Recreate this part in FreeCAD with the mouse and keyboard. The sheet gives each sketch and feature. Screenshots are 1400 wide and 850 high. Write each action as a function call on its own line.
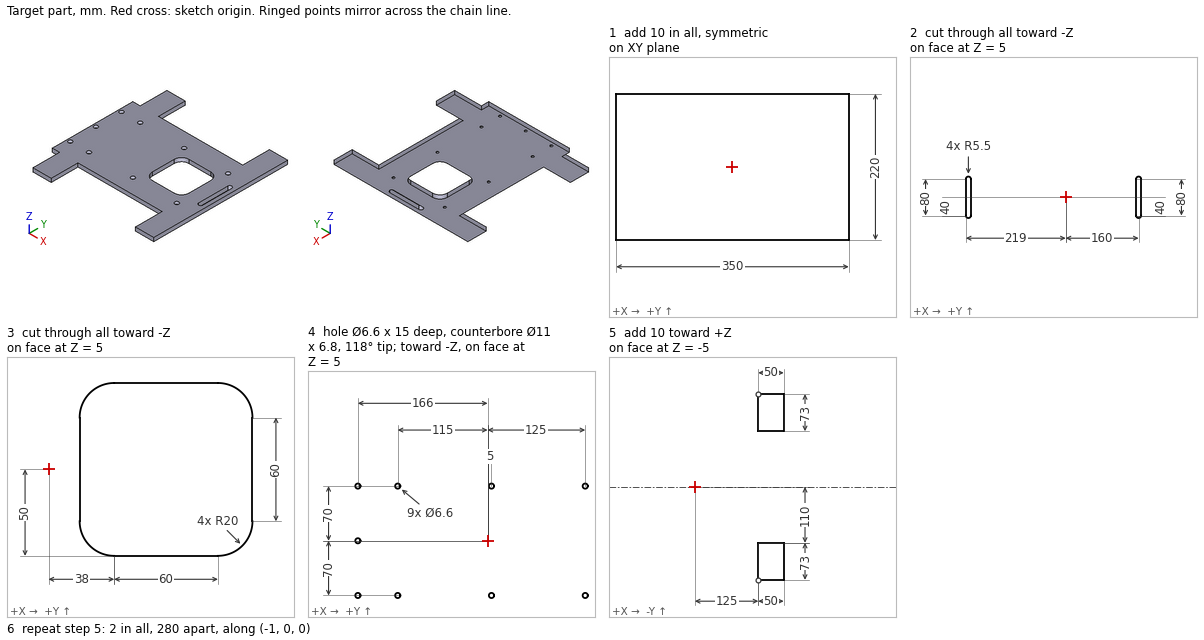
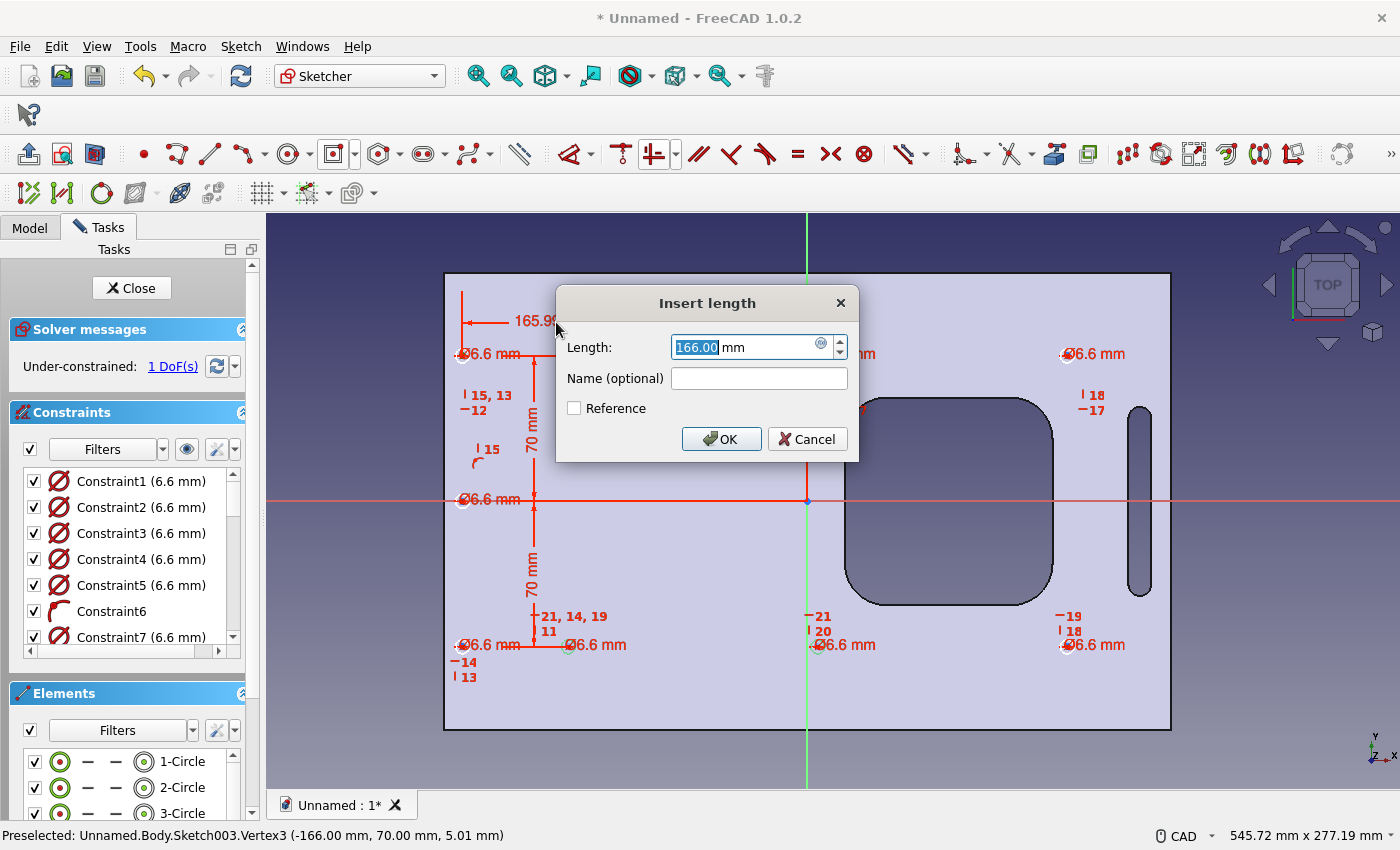
text(166)
key(Return)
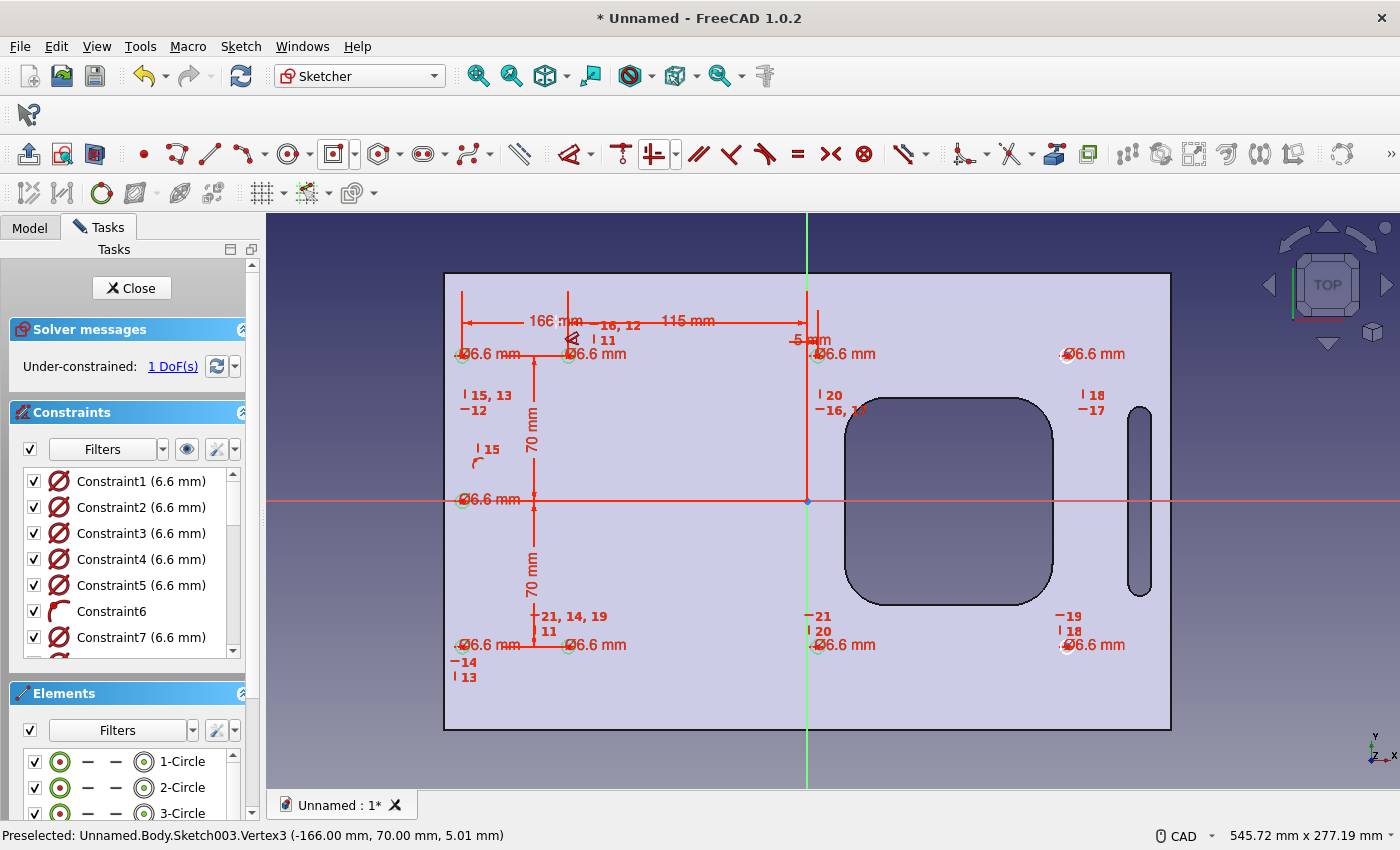
click(1067, 356)
click(937, 322)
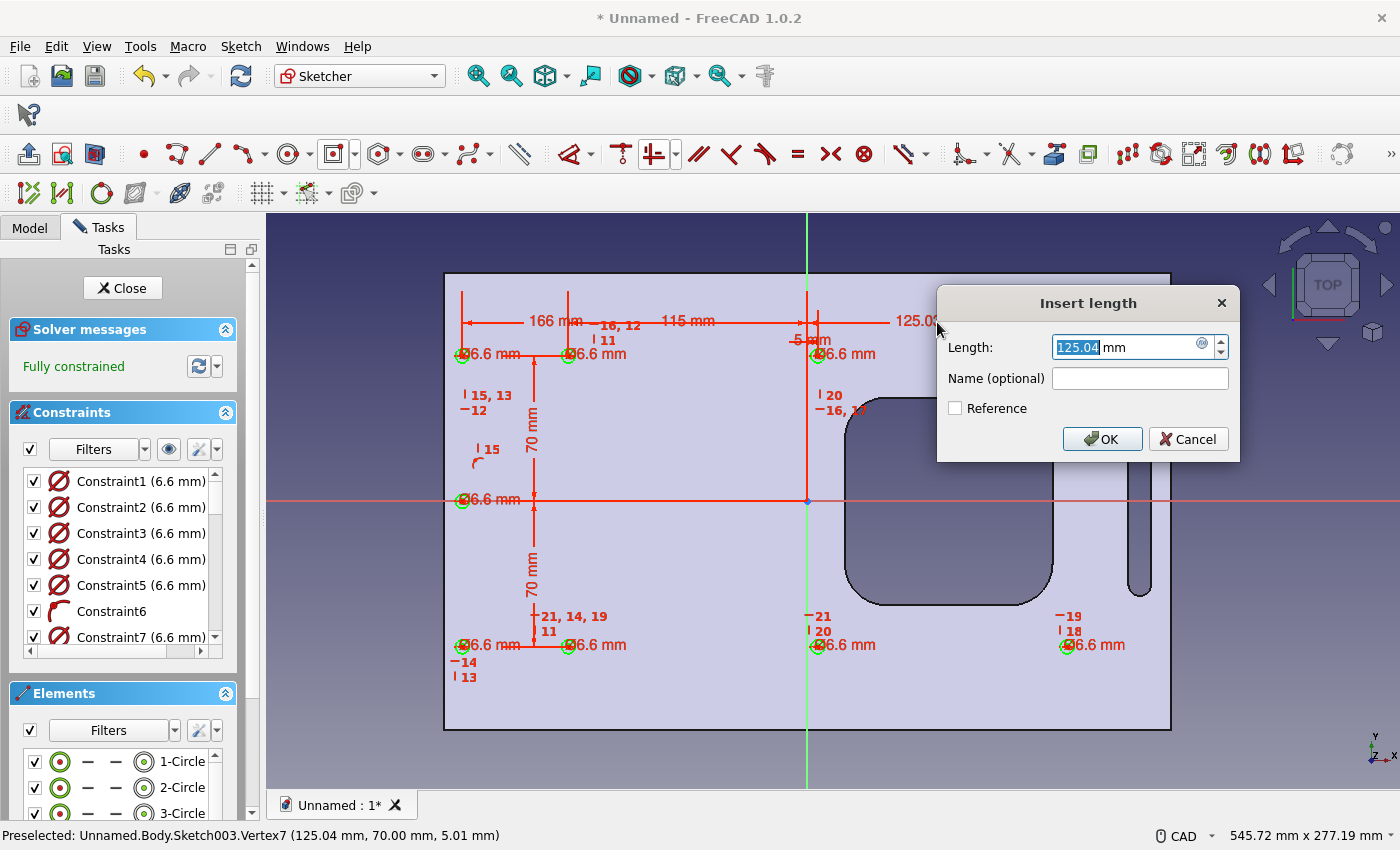
text(125)
key(Return)
key(Escape)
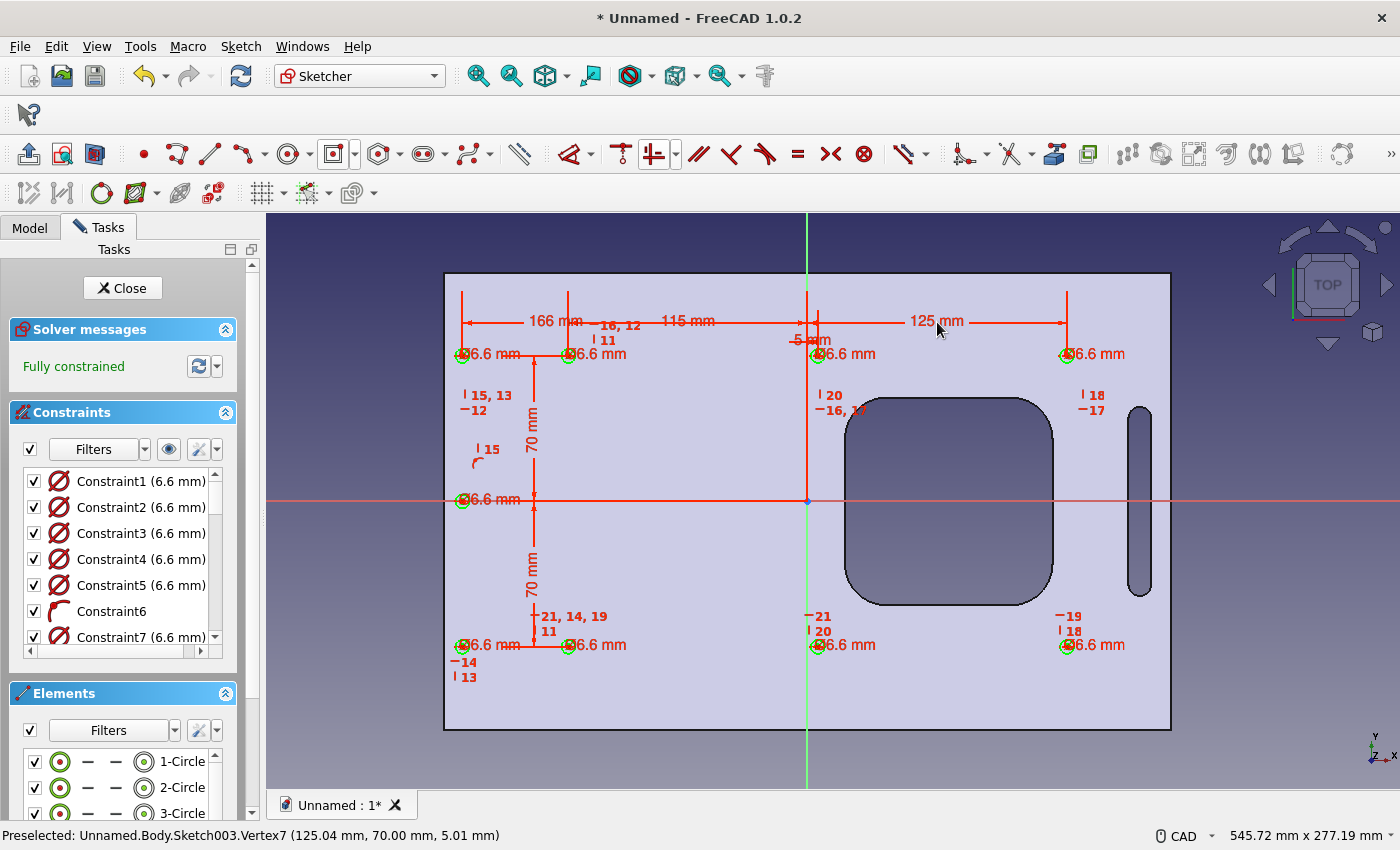
click(123, 288)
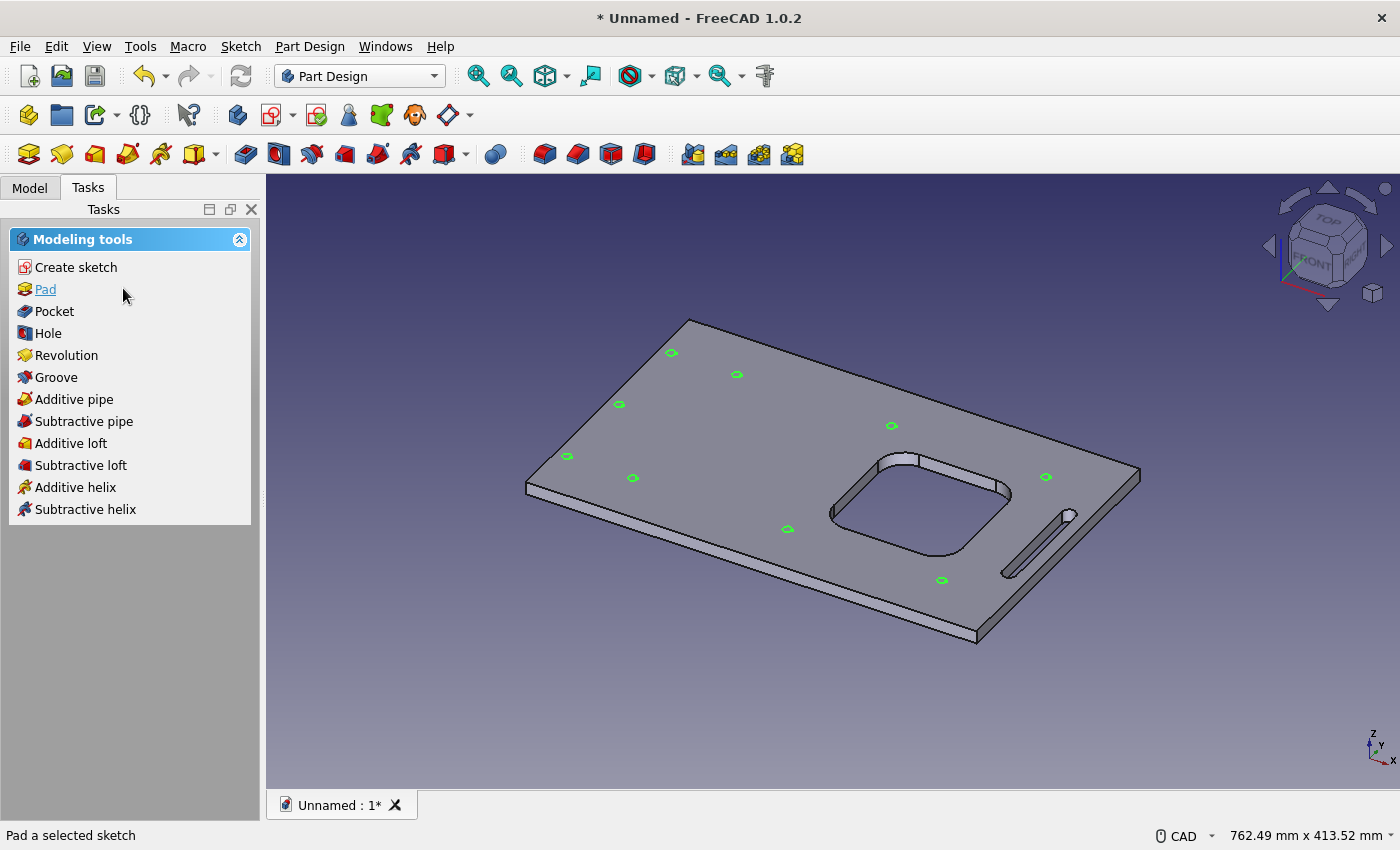
click(279, 154)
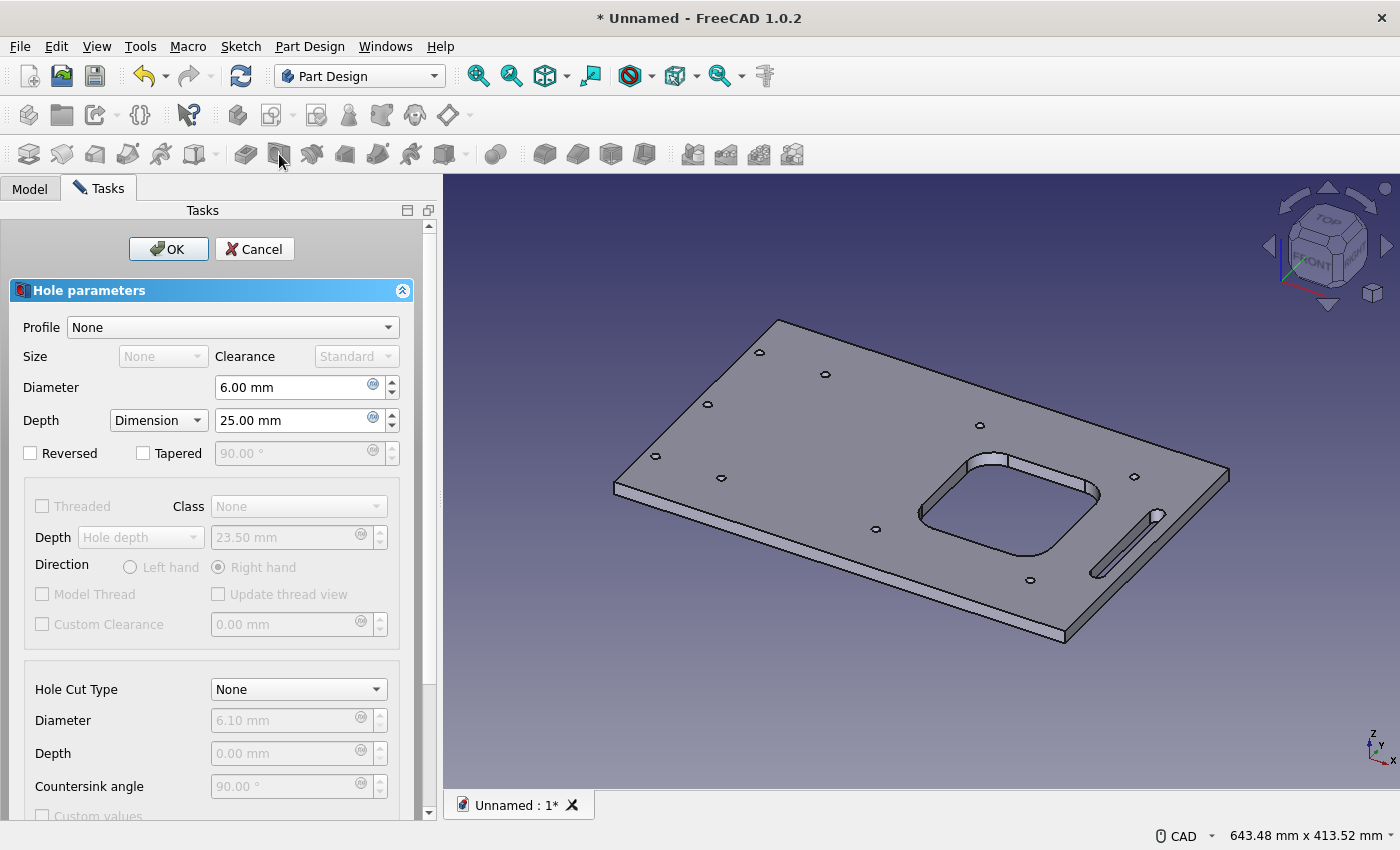
triple_click(300, 388)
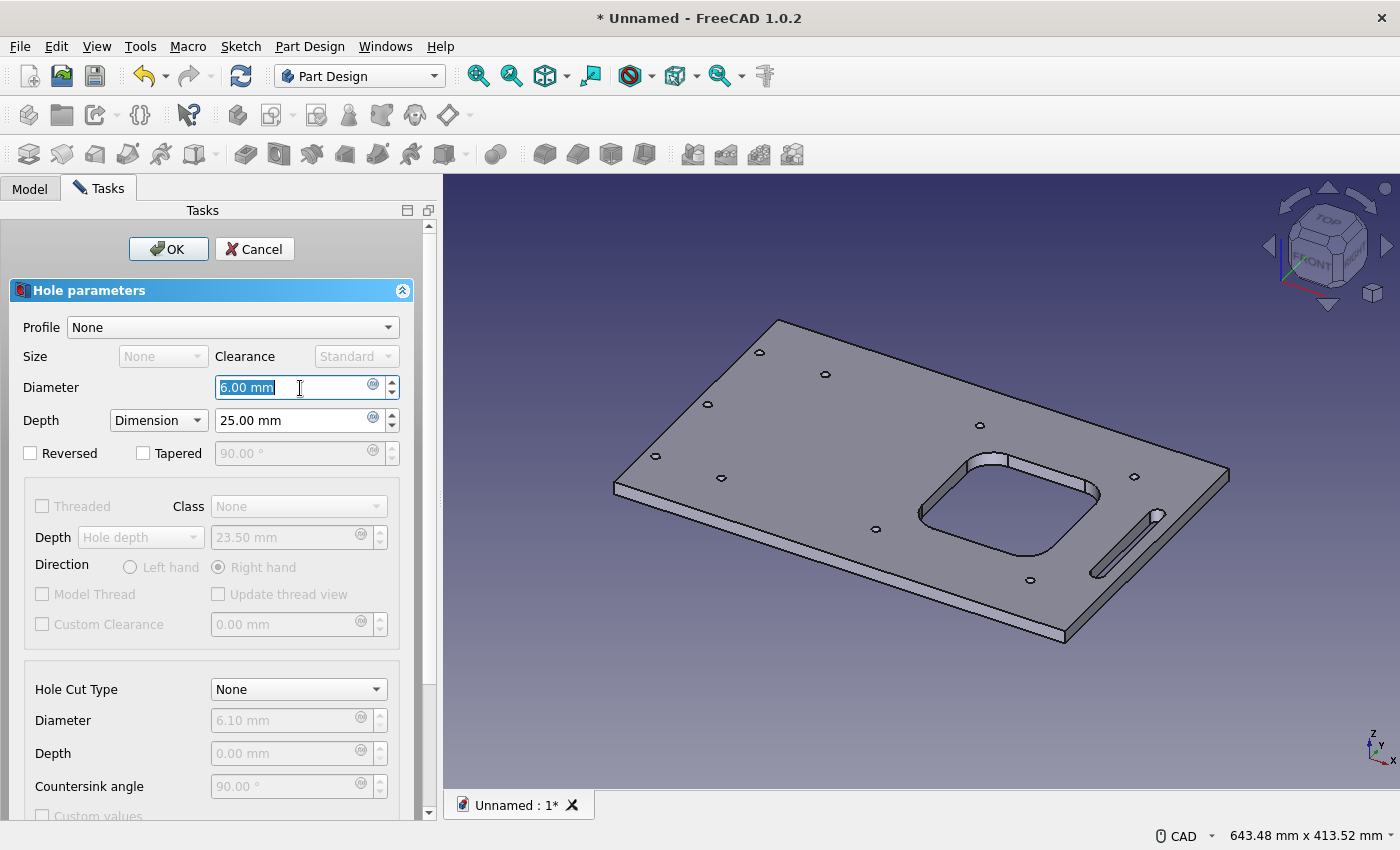
text(6.6)
key(Tab)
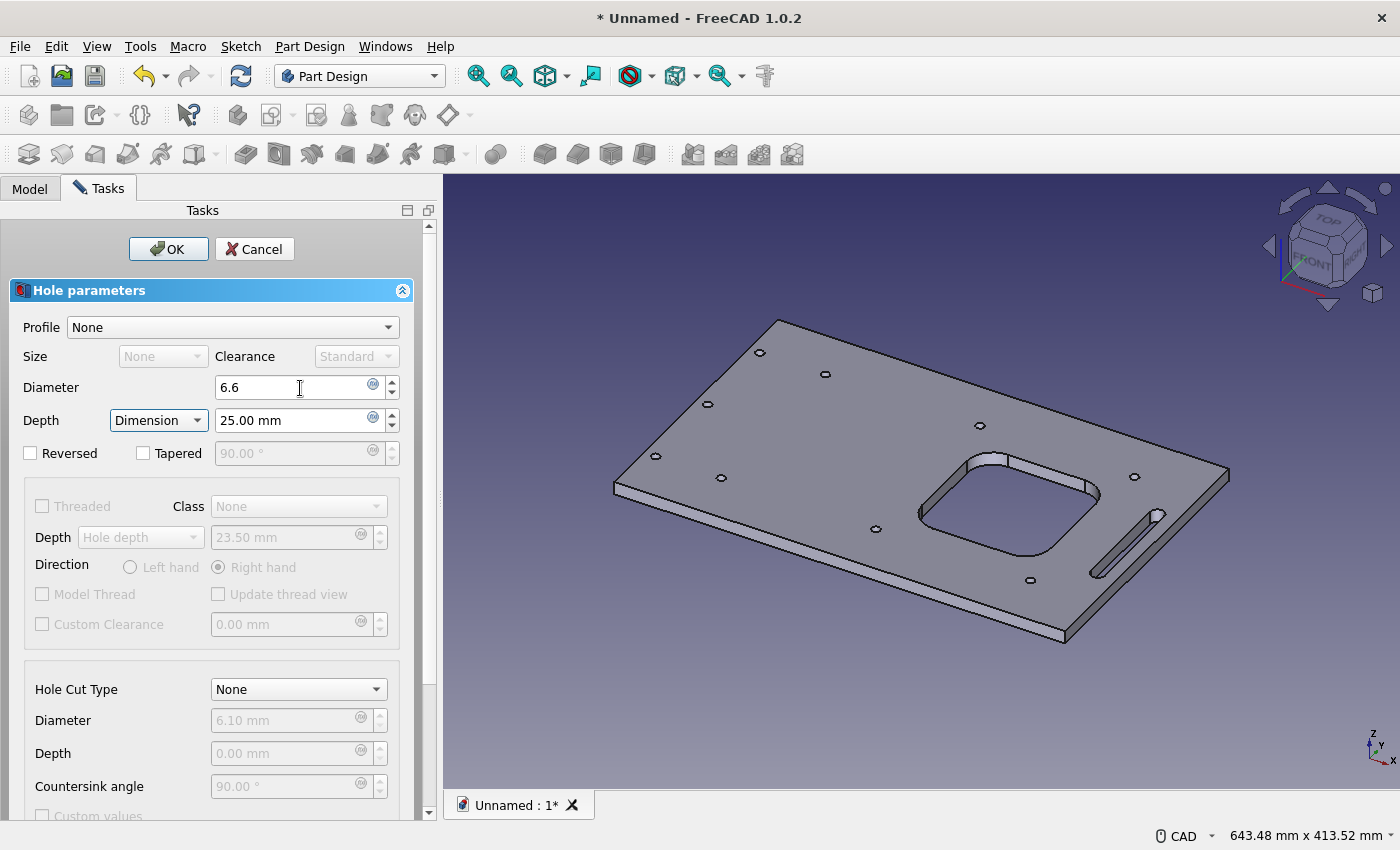
triple_click(300, 420)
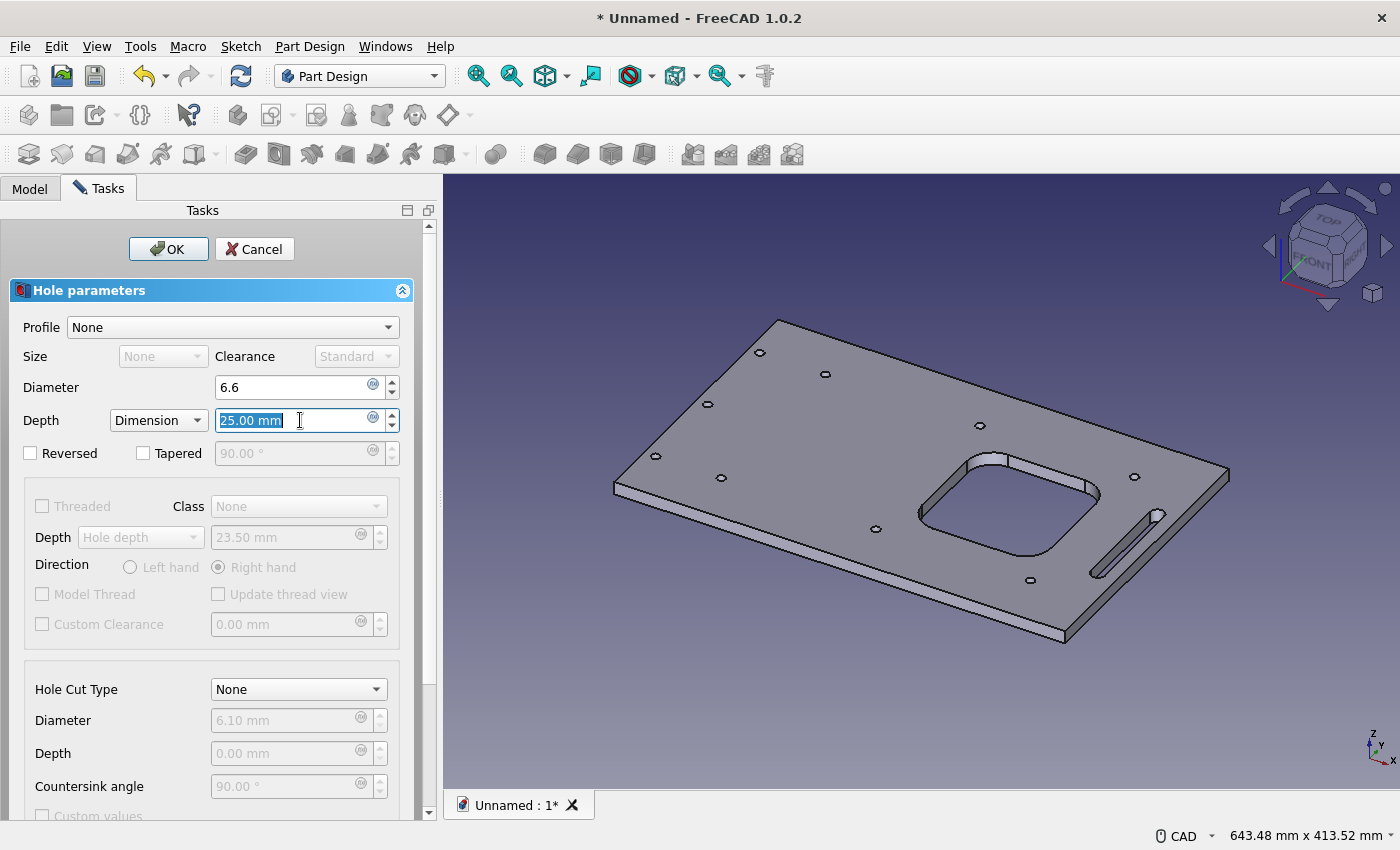
text(15)
key(Tab)